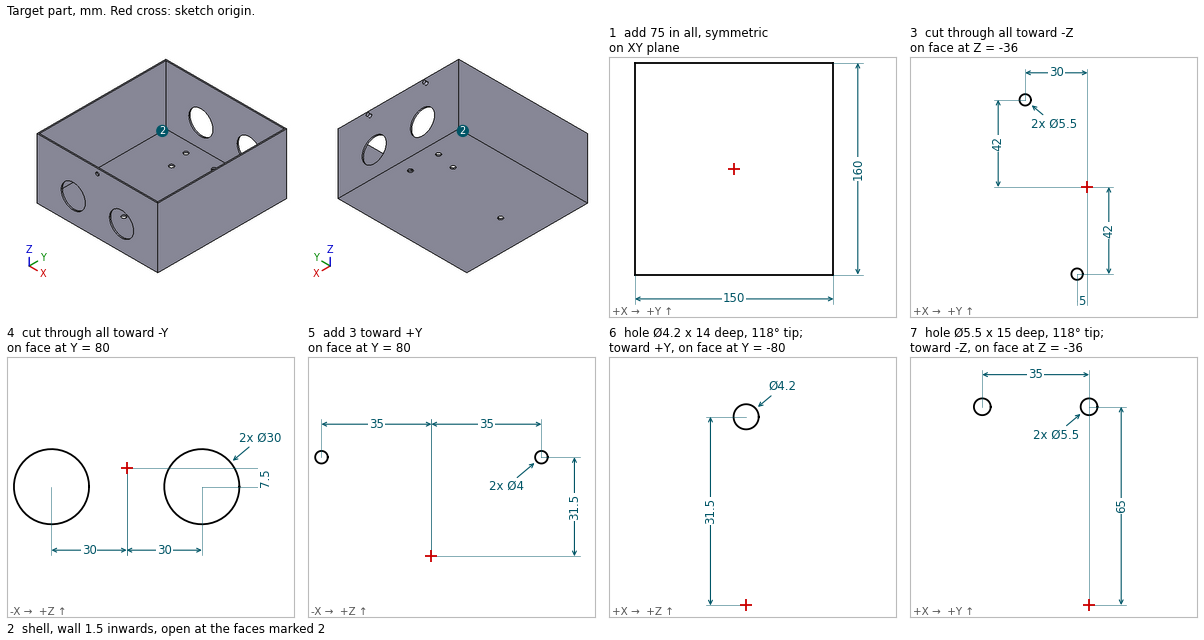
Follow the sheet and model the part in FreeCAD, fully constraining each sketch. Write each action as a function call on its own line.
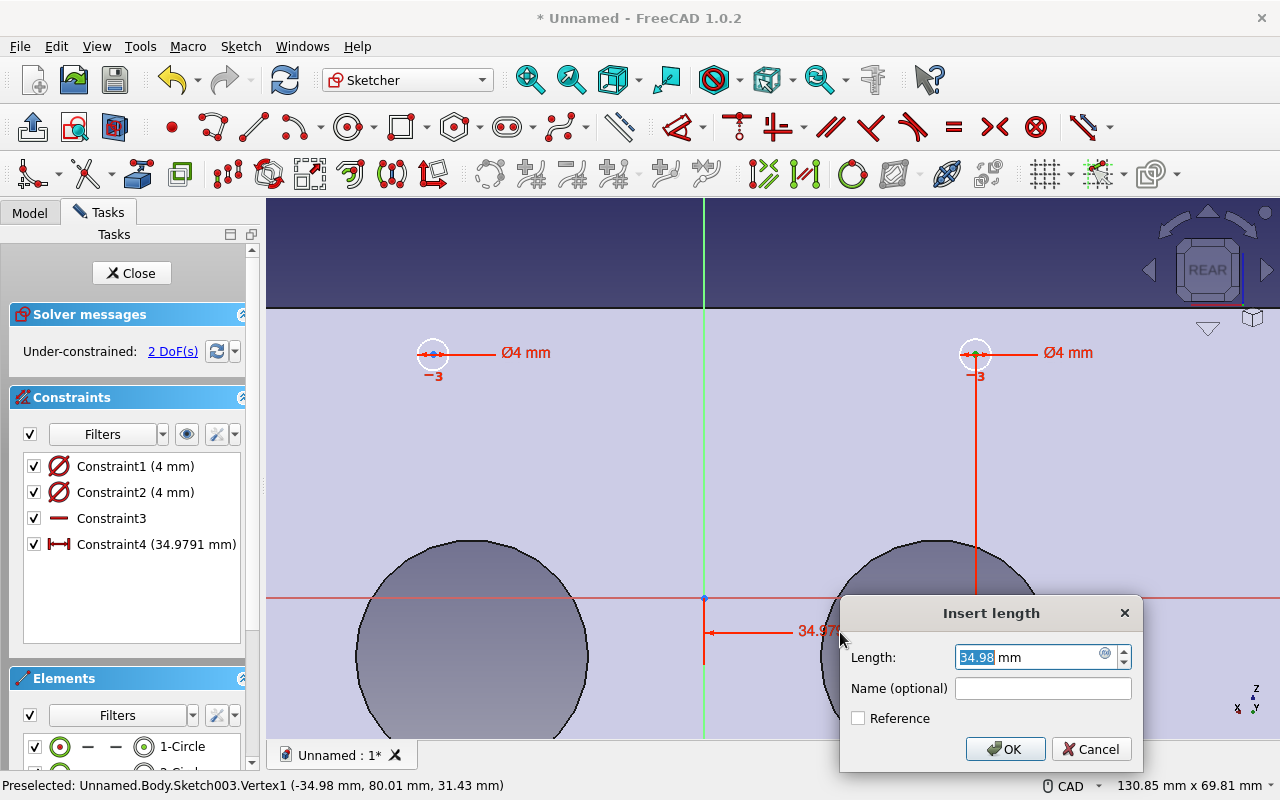
text(35)
key(Return)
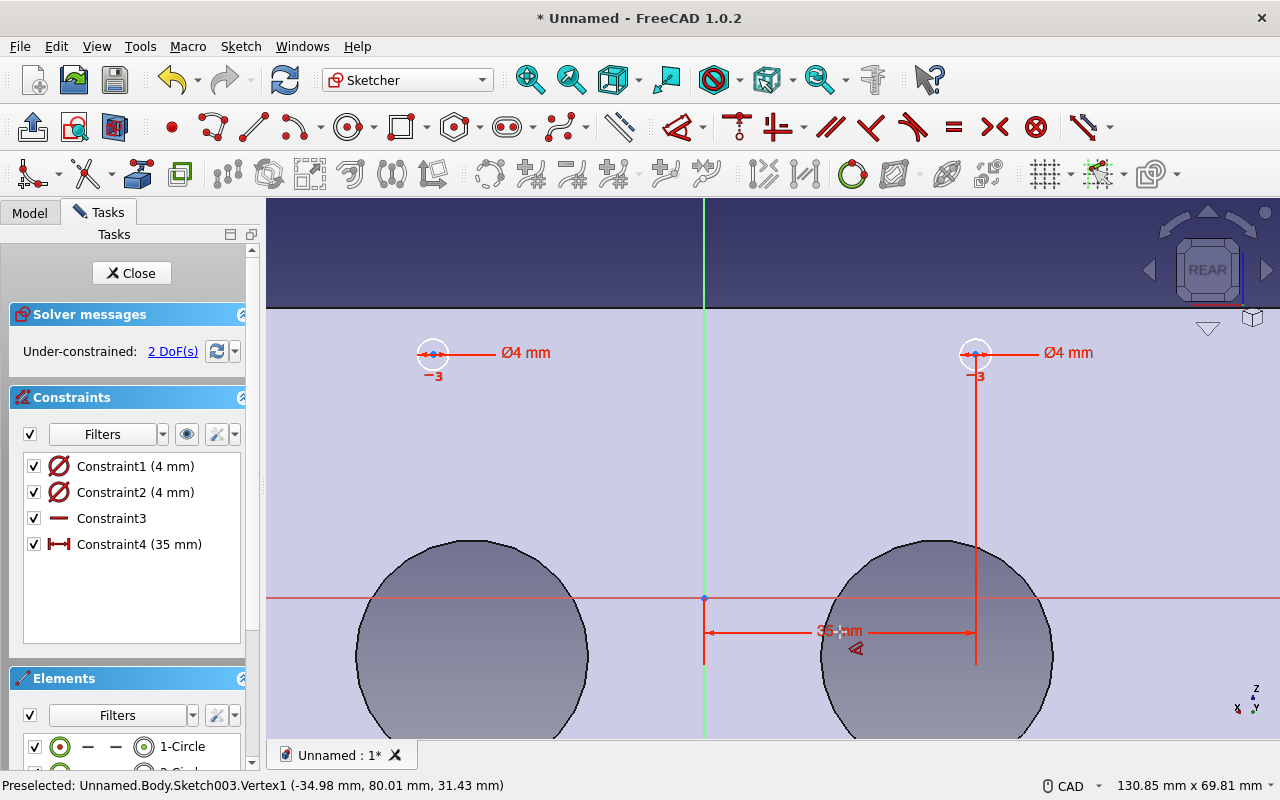
click(433, 355)
click(569, 632)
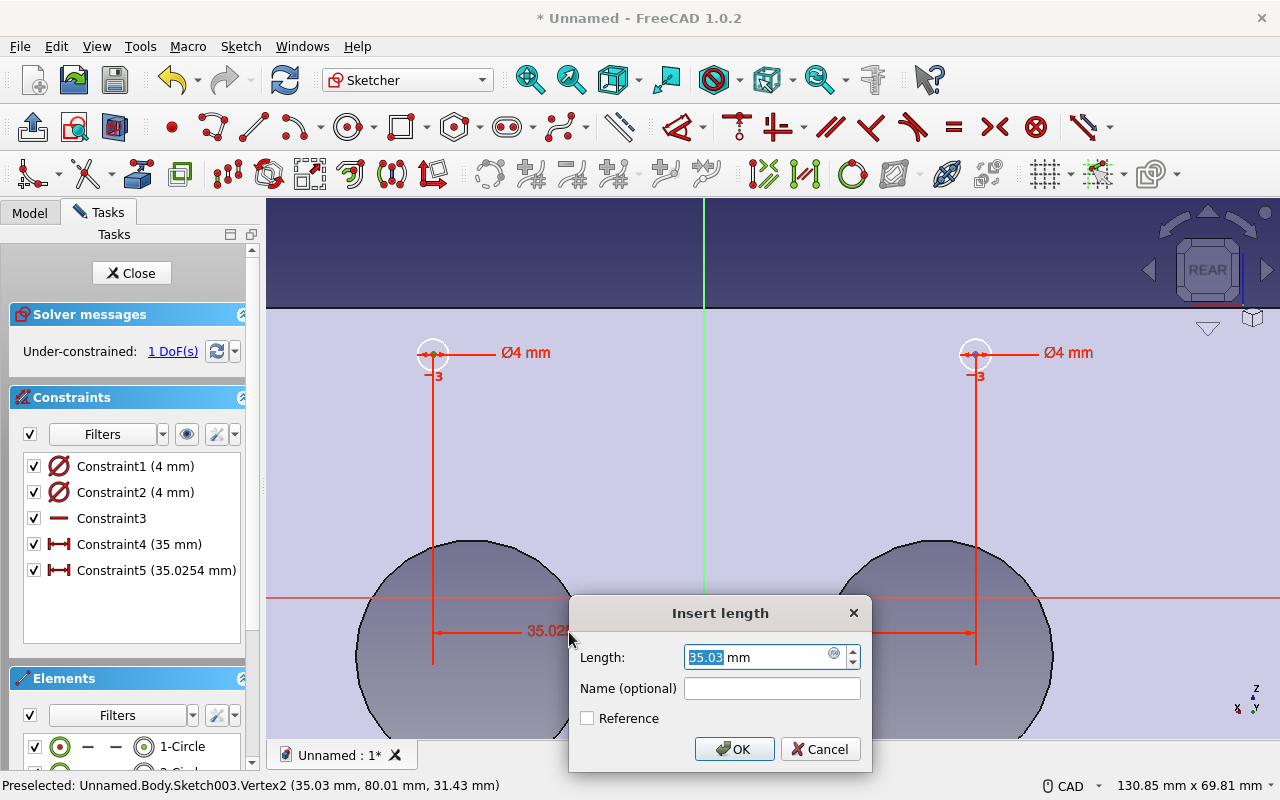
text(35)
key(Return)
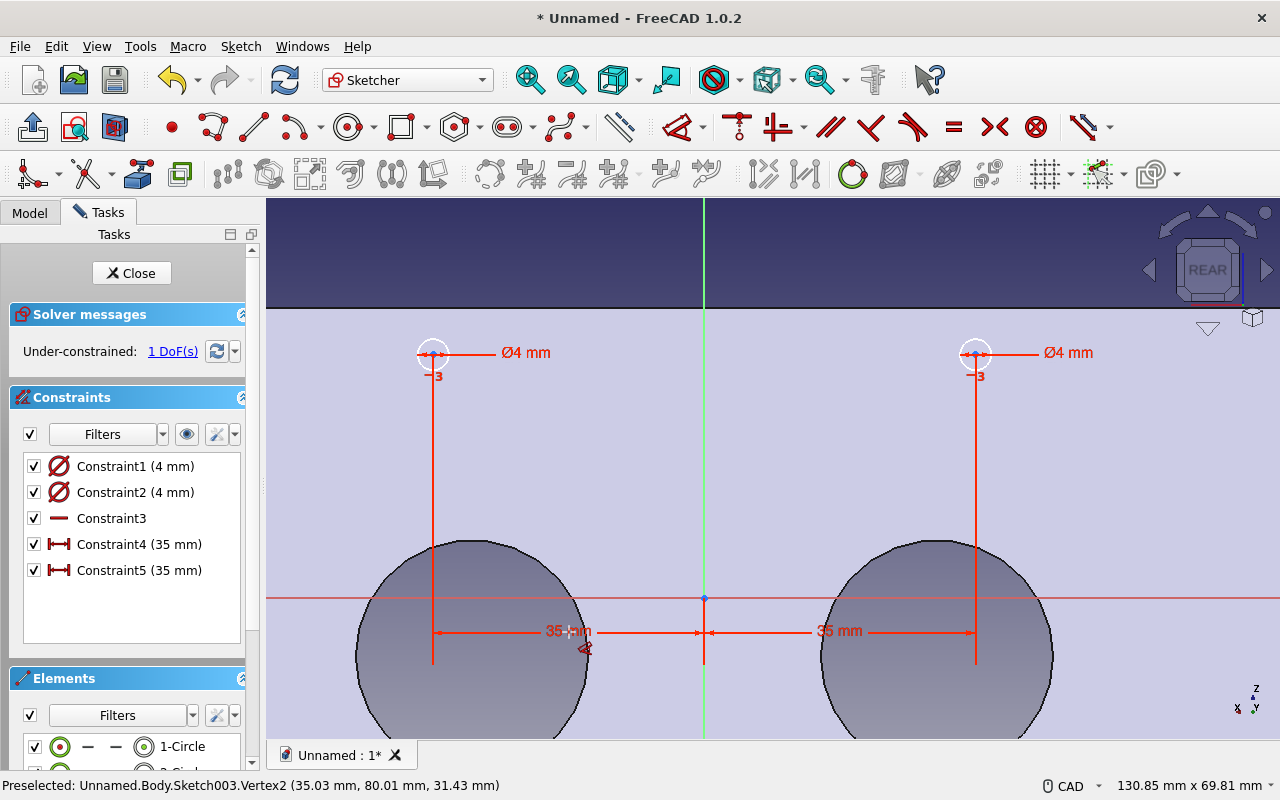
click(976, 355)
click(1010, 477)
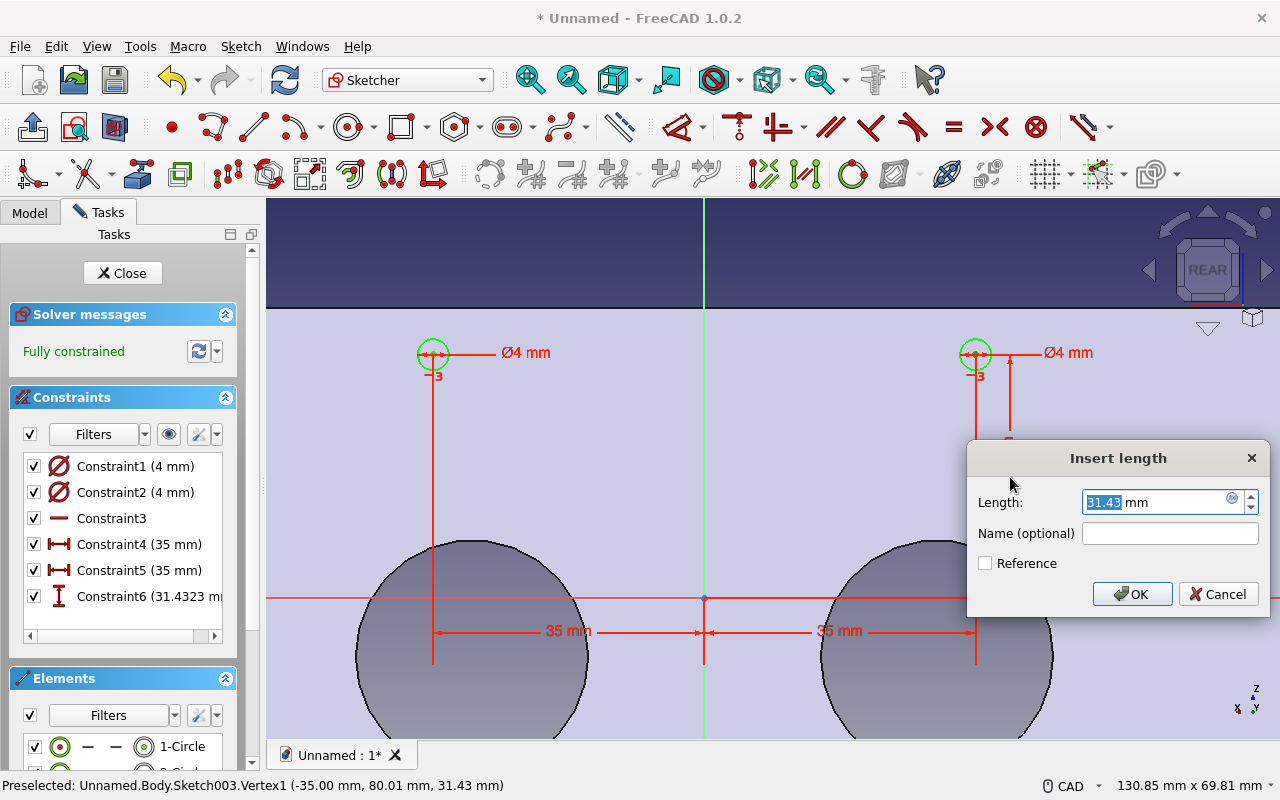
text(31.5)
key(Return)
key(Escape)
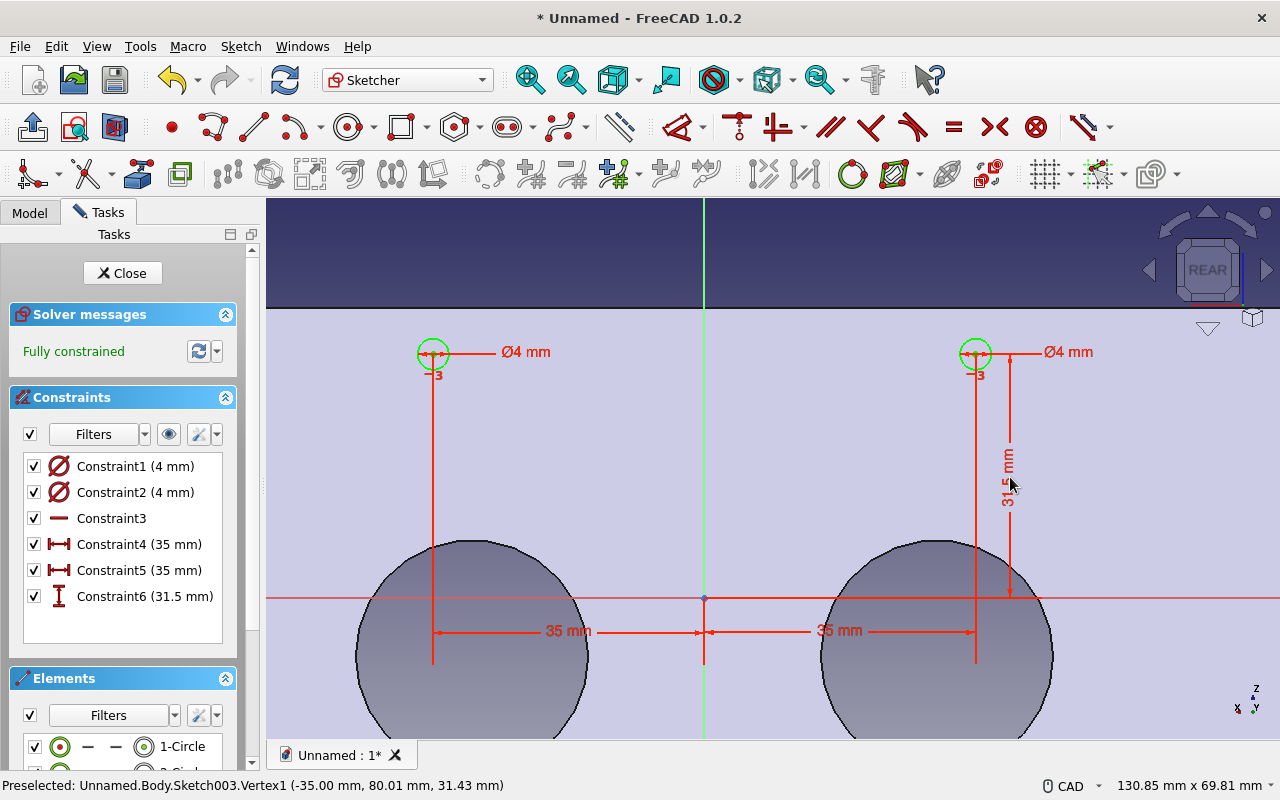
click(123, 273)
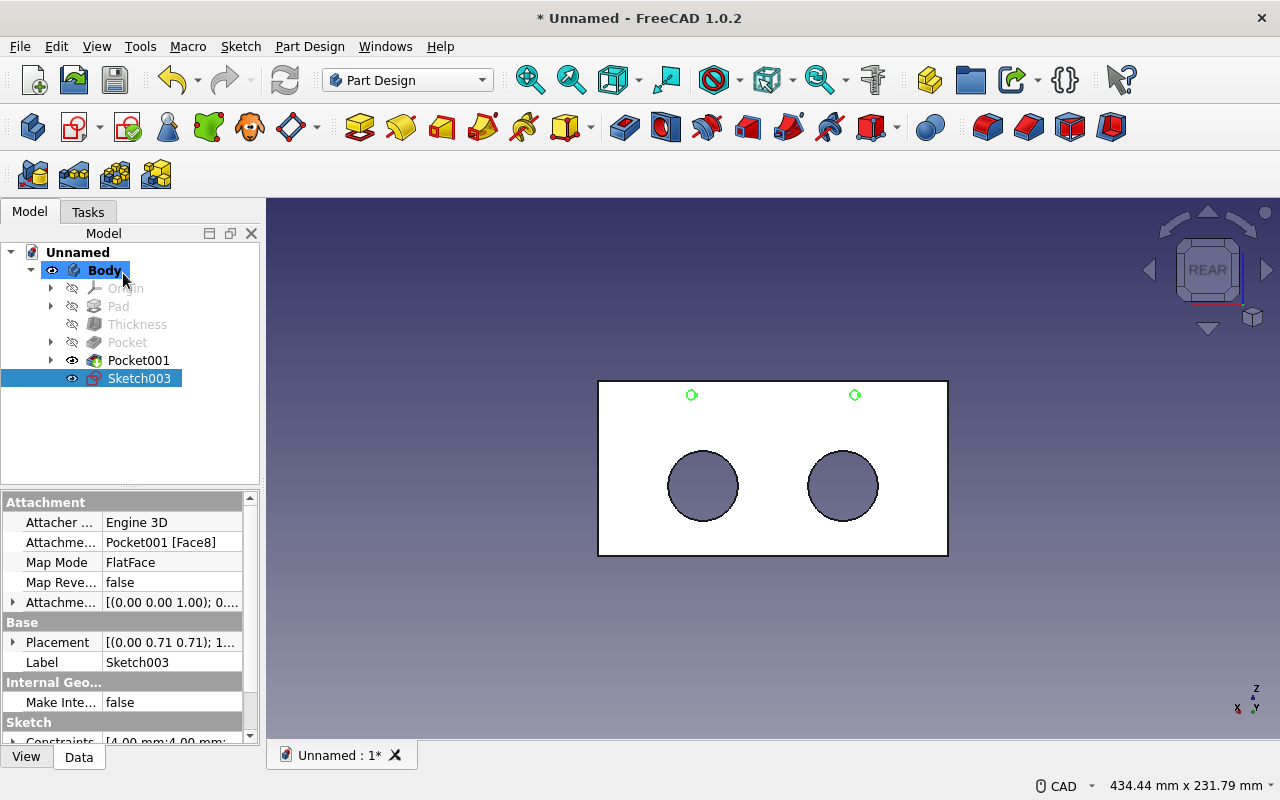
click(360, 128)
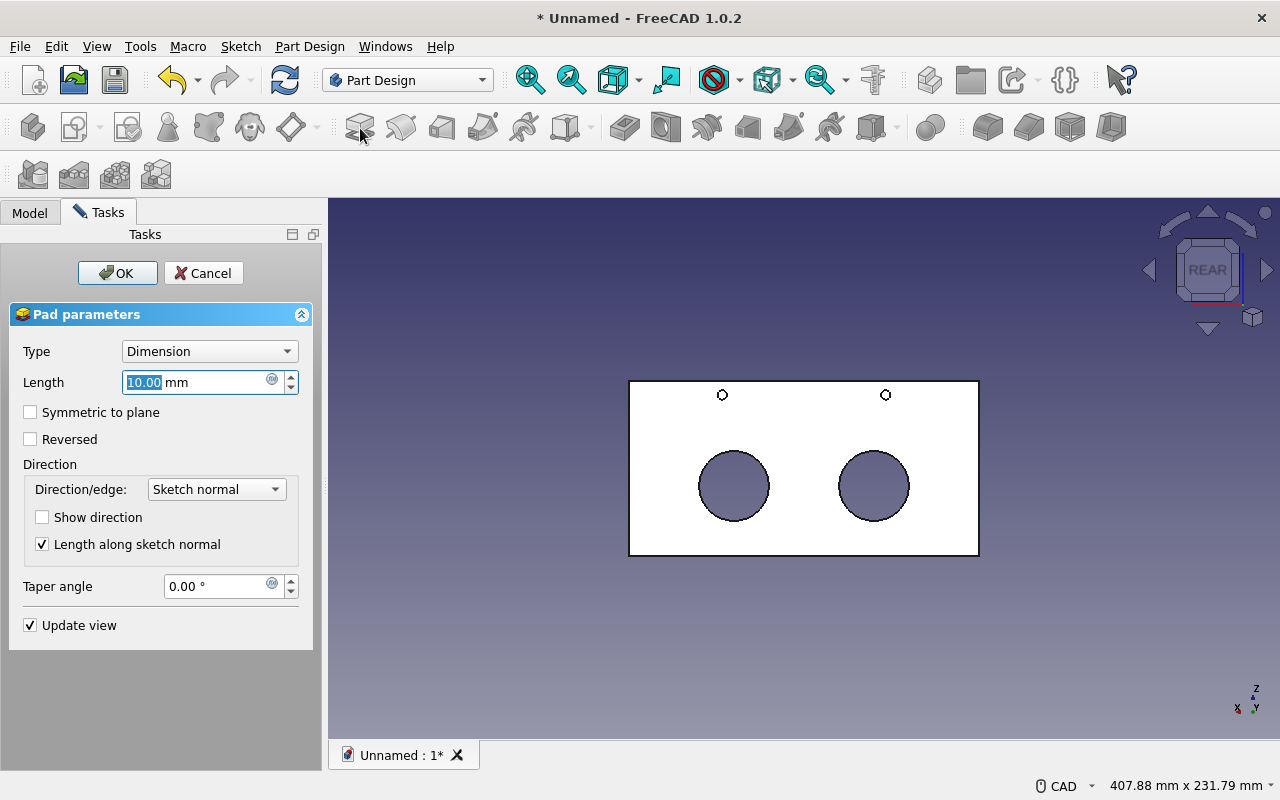
text(3)
key(Tab)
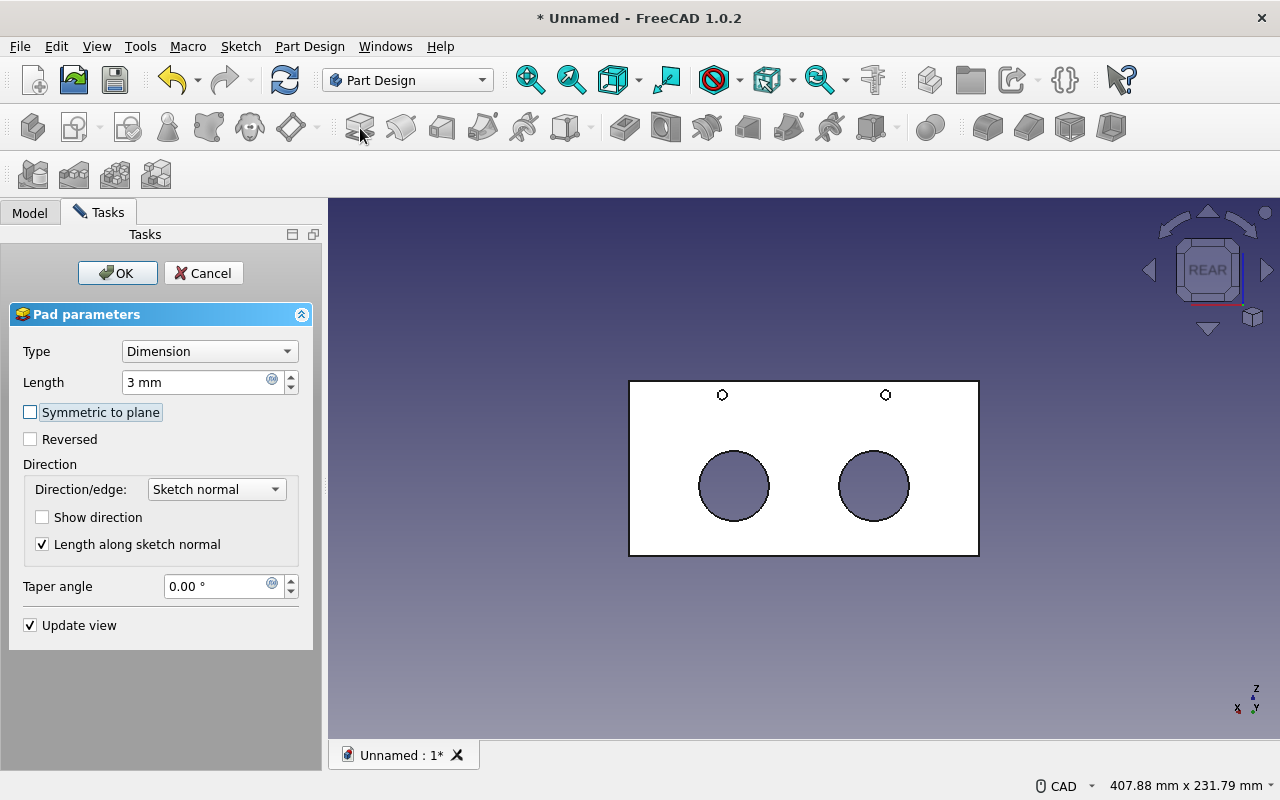
click(118, 273)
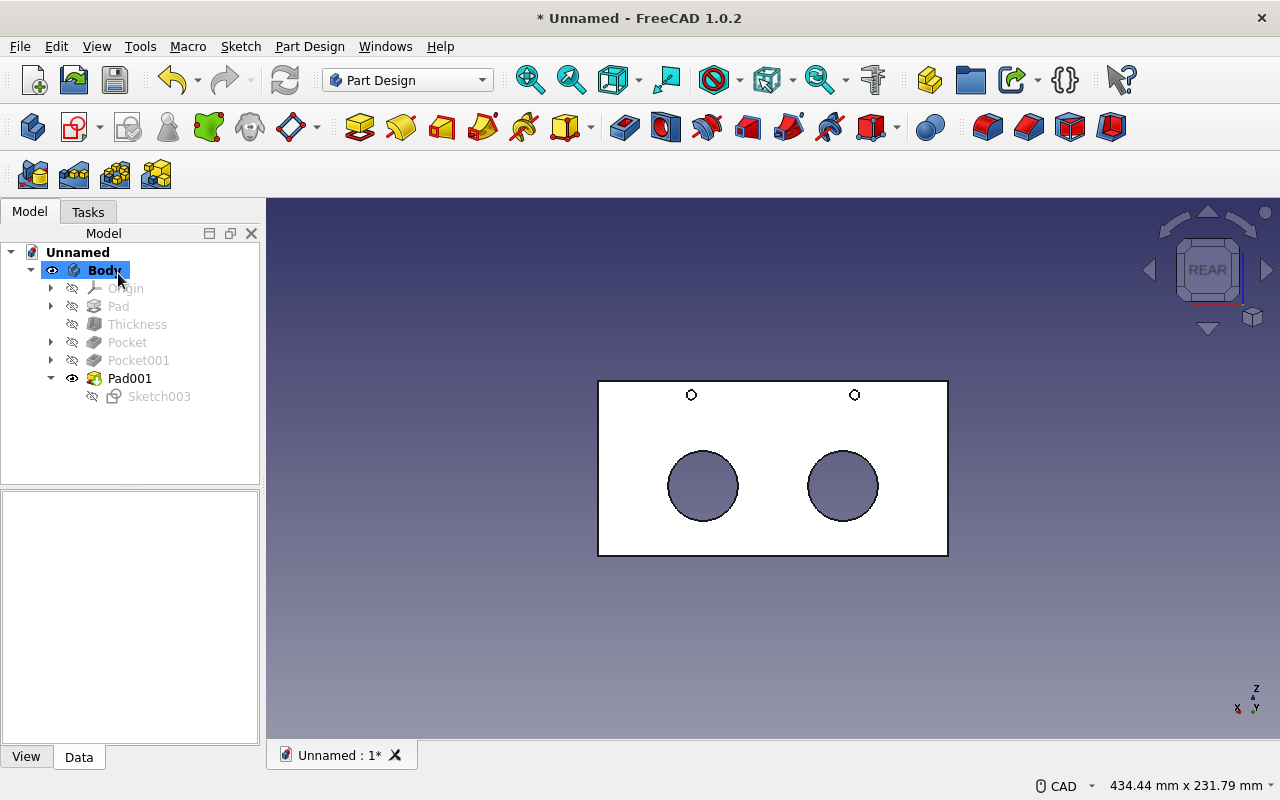
key(v)
key(f)